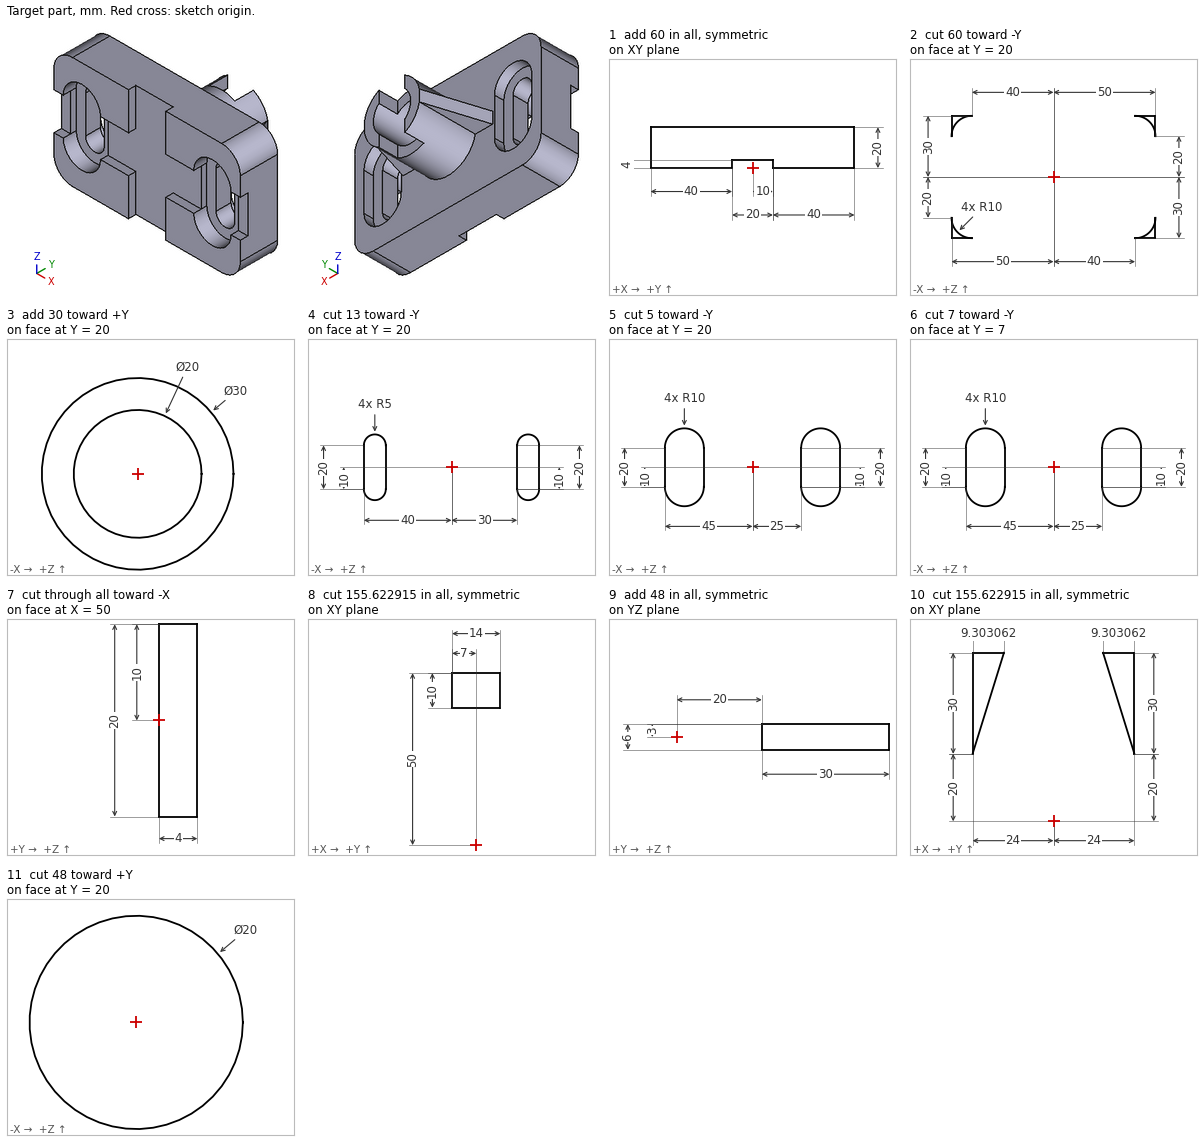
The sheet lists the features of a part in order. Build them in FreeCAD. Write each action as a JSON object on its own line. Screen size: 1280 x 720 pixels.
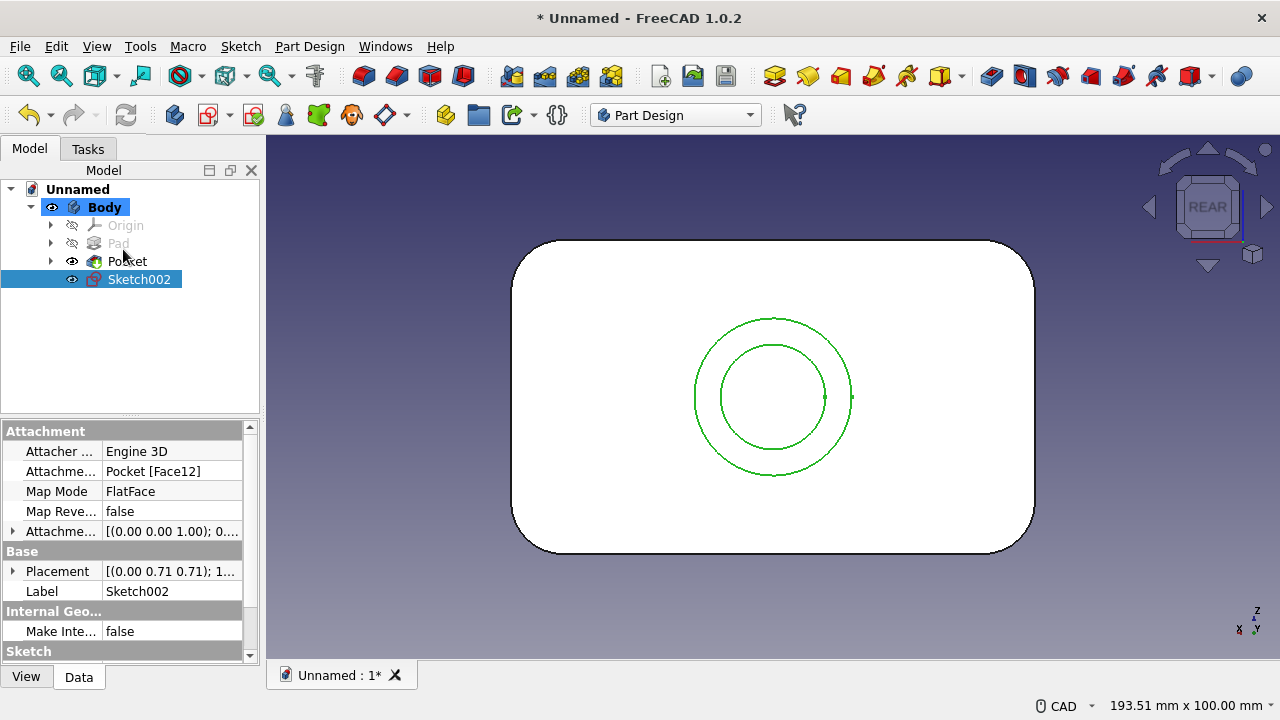
{"action": "left_click", "coordinate": [775, 76]}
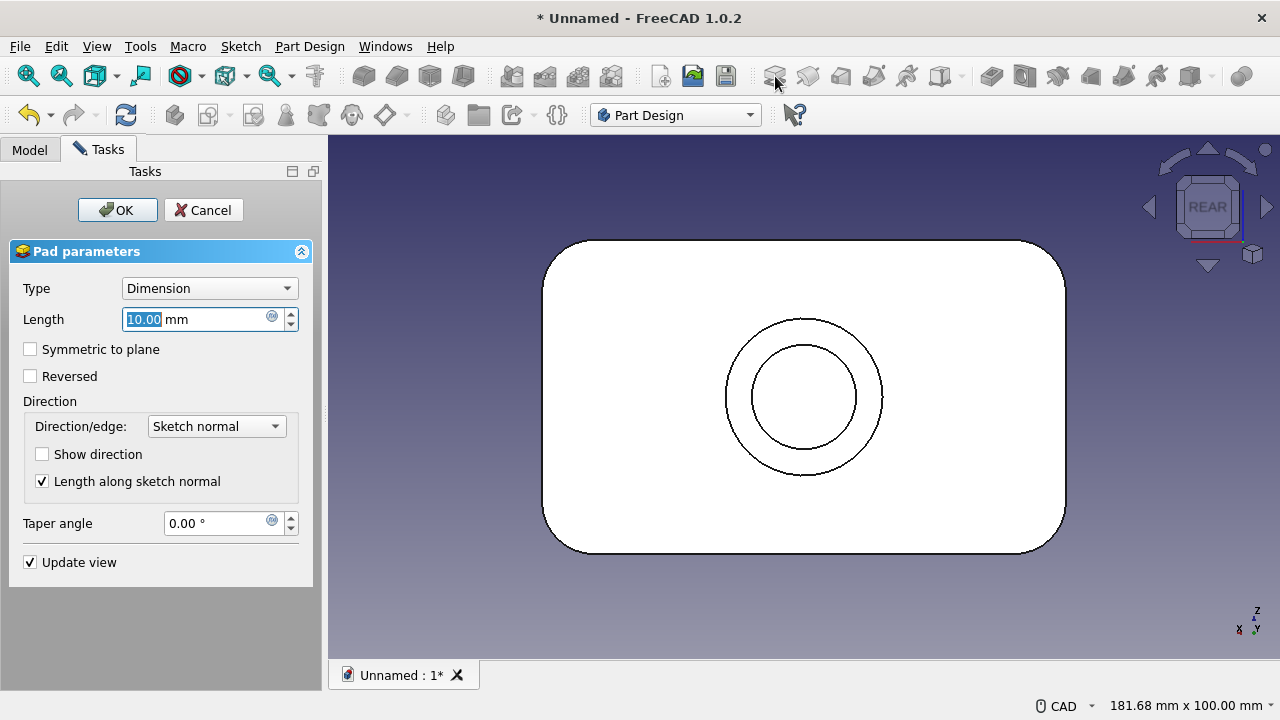
{"action": "type", "text": "30"}
{"action": "key", "text": "Tab"}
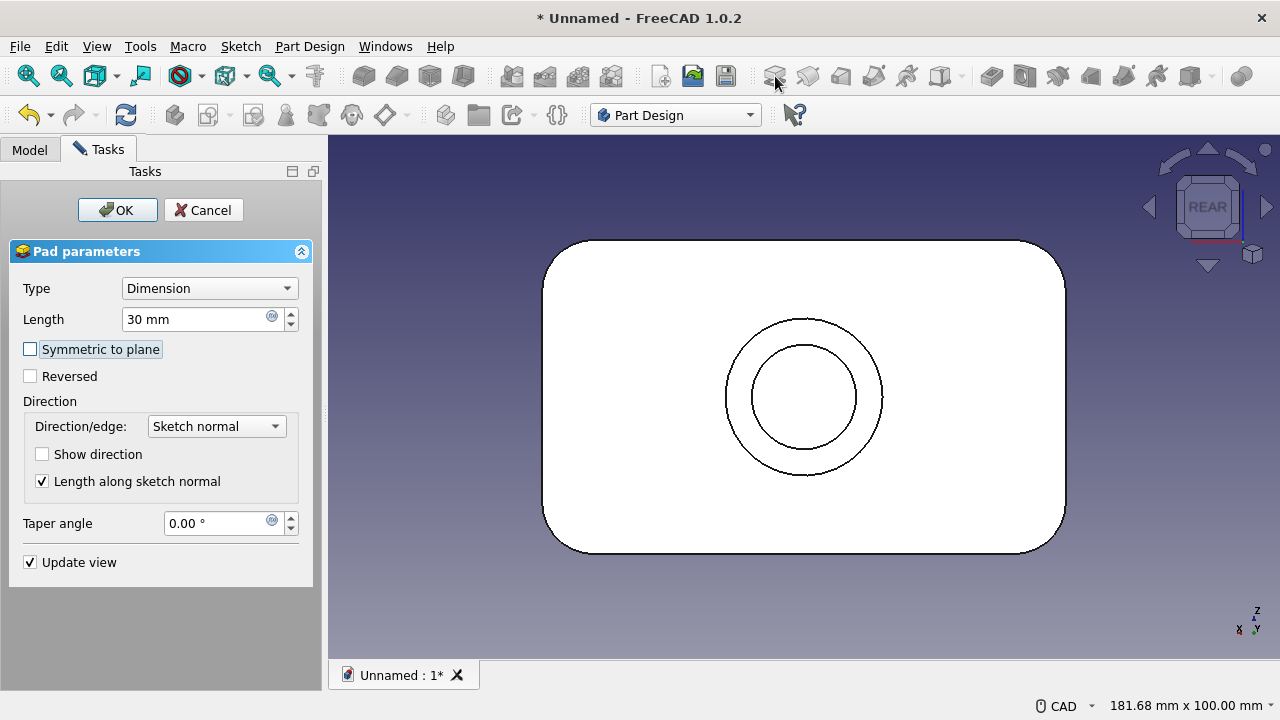
{"action": "left_click", "coordinate": [118, 210]}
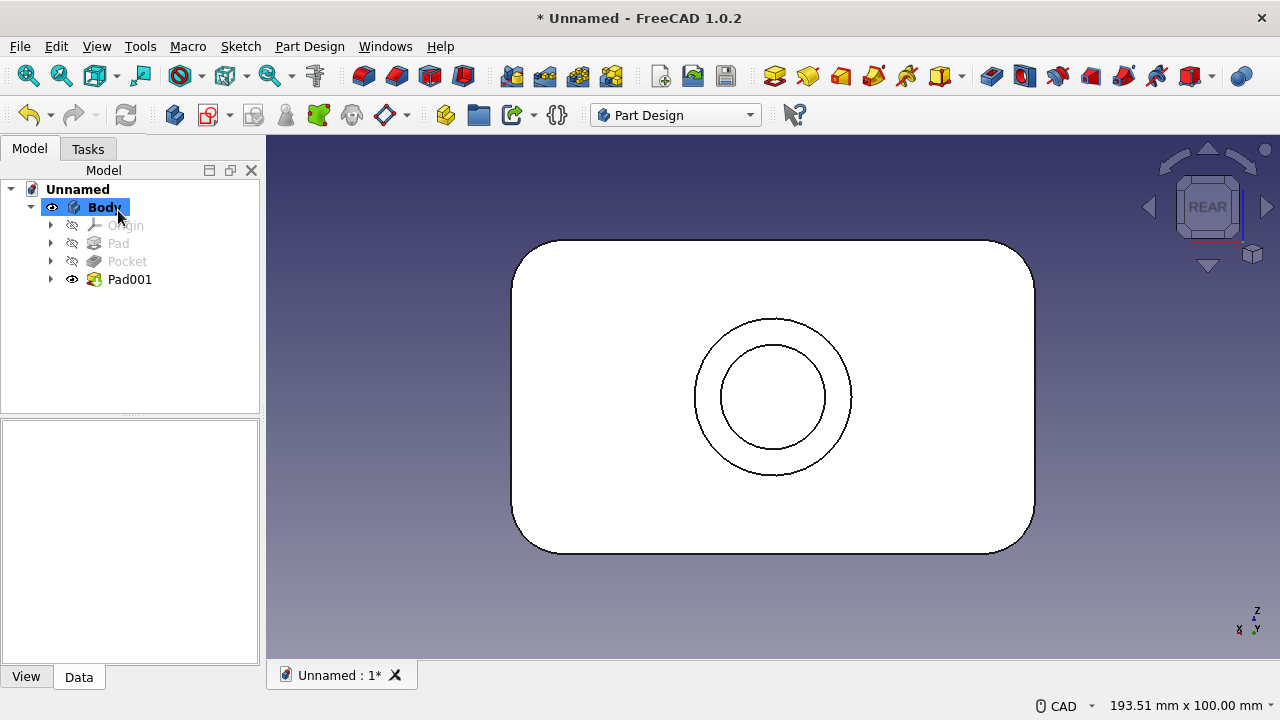
{"action": "left_click", "coordinate": [623, 351]}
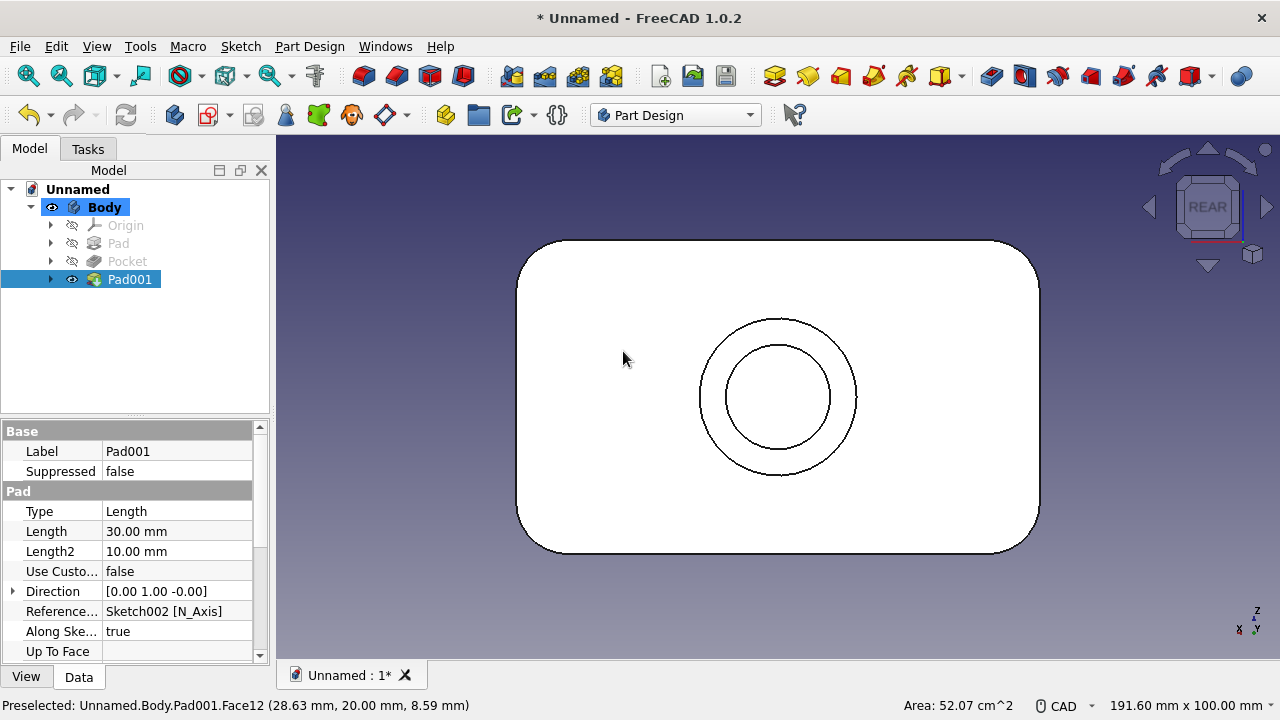
{"action": "left_click", "coordinate": [208, 116]}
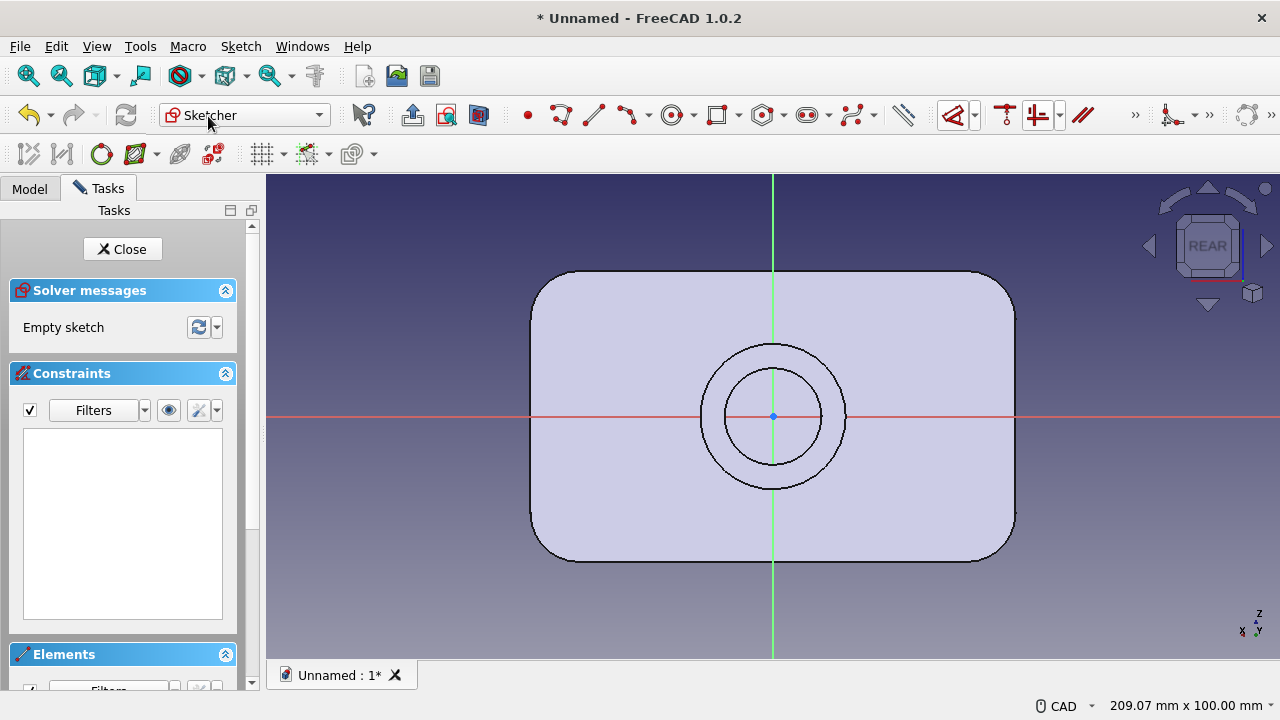
{"action": "key", "text": "q s"}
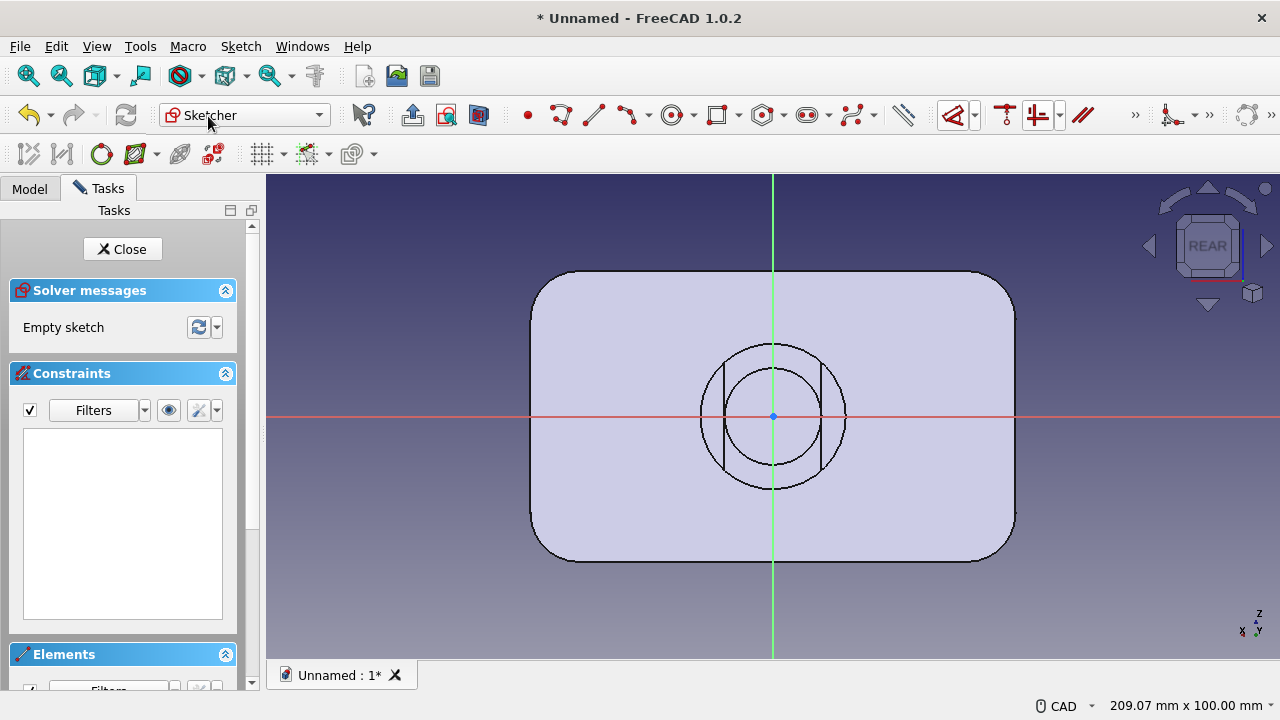
{"action": "scroll", "coordinate": [912, 417], "scroll_direction": "up", "scroll_amount": 2}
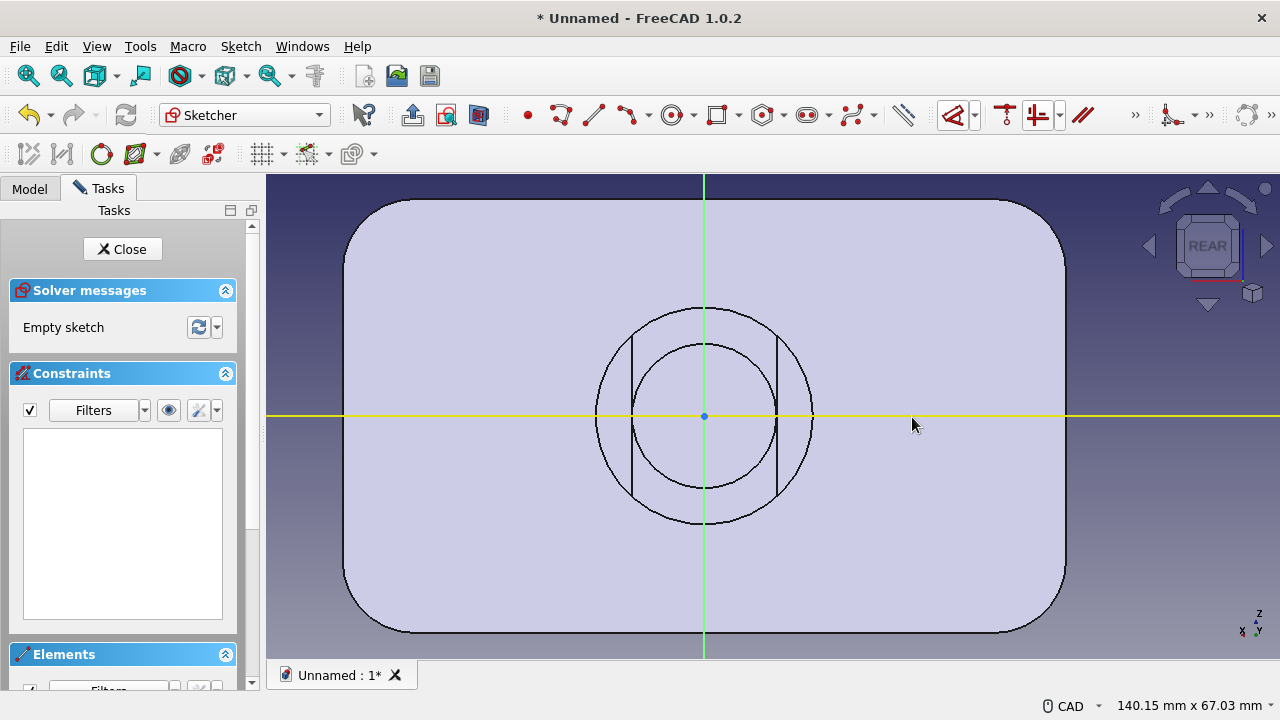
{"action": "key", "text": "g s"}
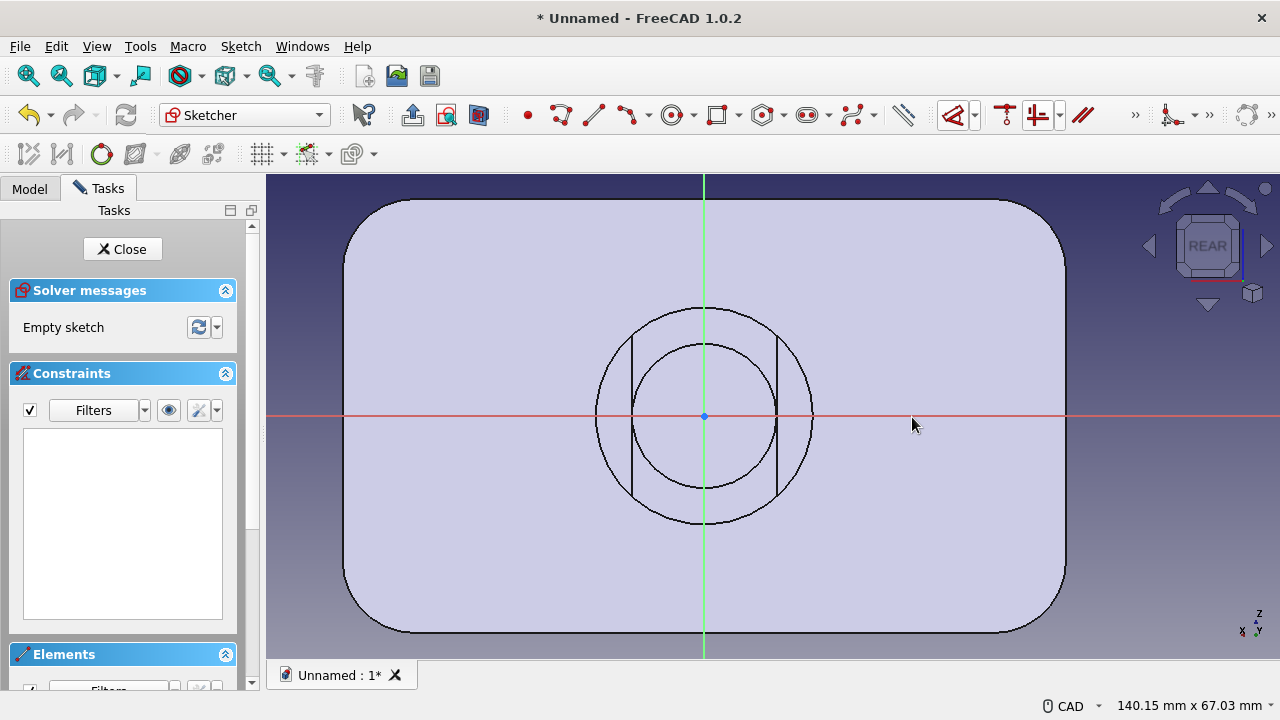
{"action": "left_click", "coordinate": [451, 488]}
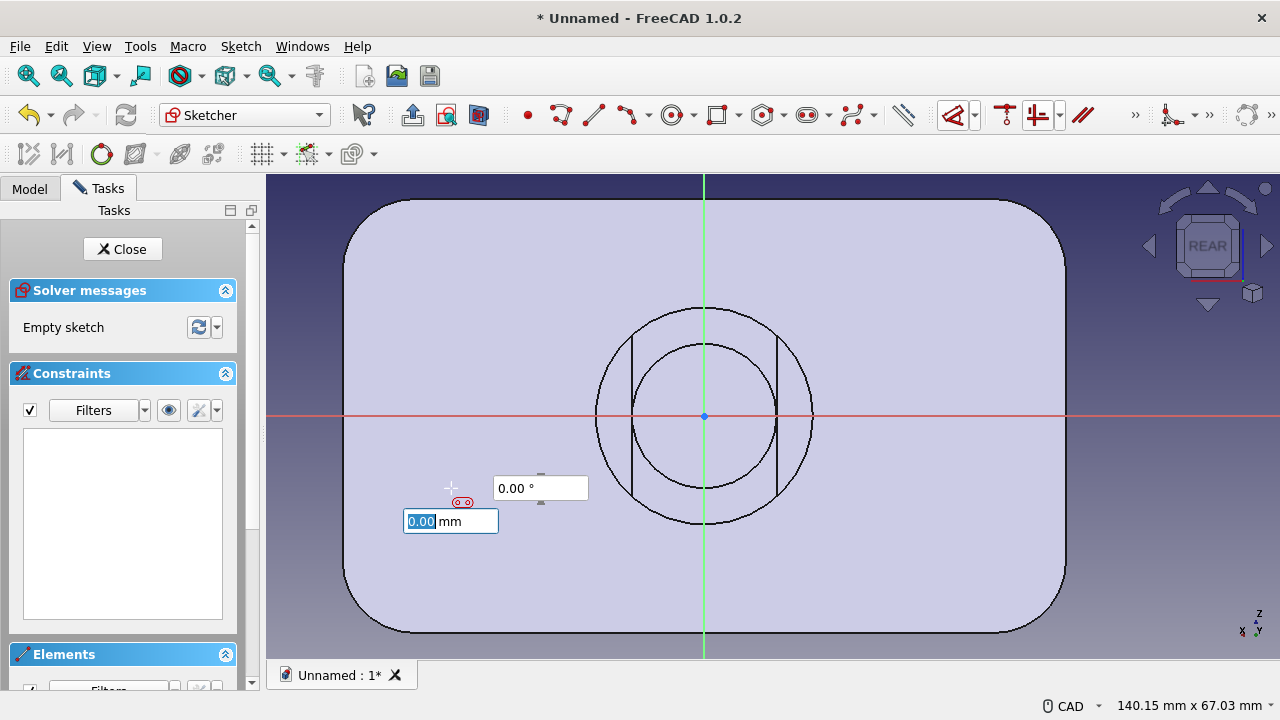
{"action": "left_click", "coordinate": [451, 344]}